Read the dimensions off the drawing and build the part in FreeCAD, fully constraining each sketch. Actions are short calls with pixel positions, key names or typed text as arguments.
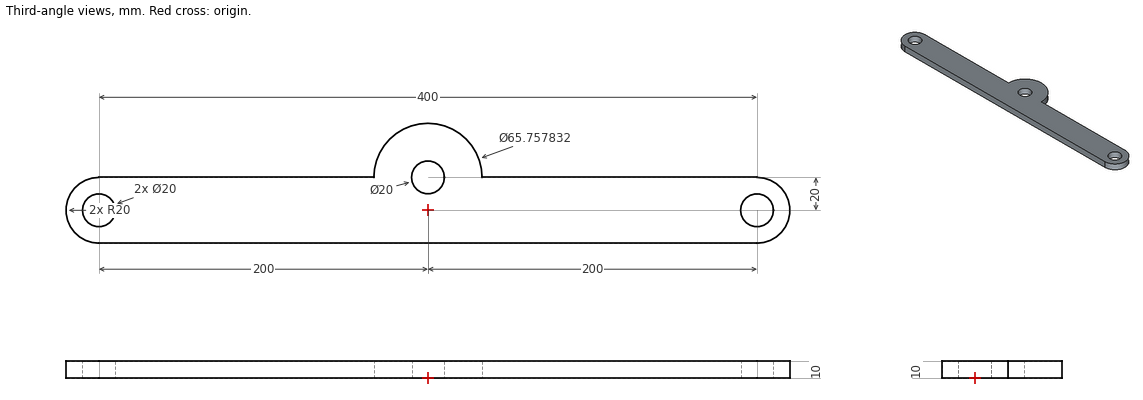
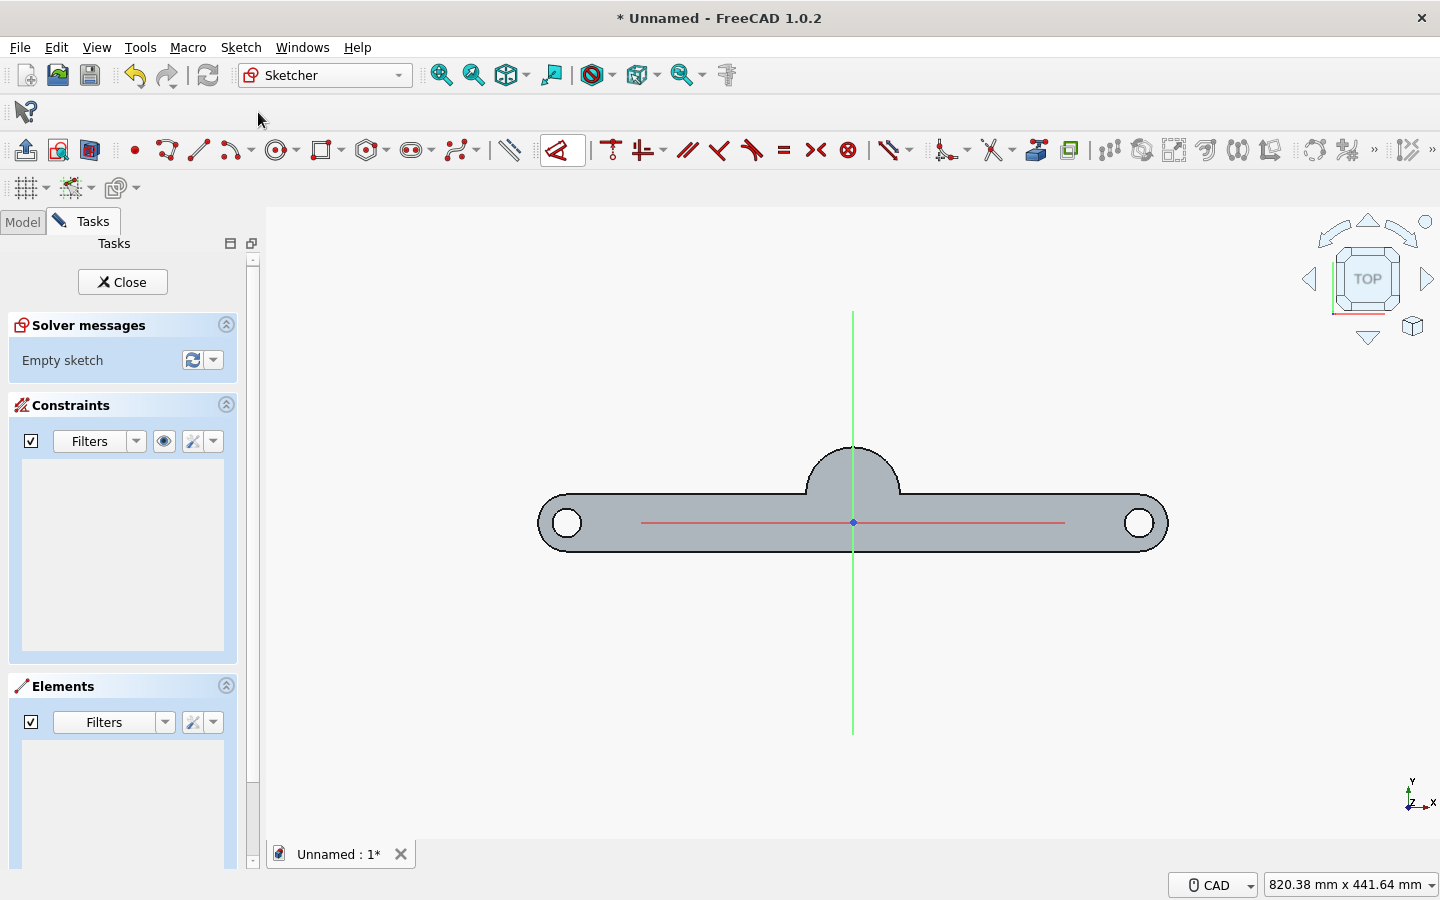
scroll(862, 499, up, 11)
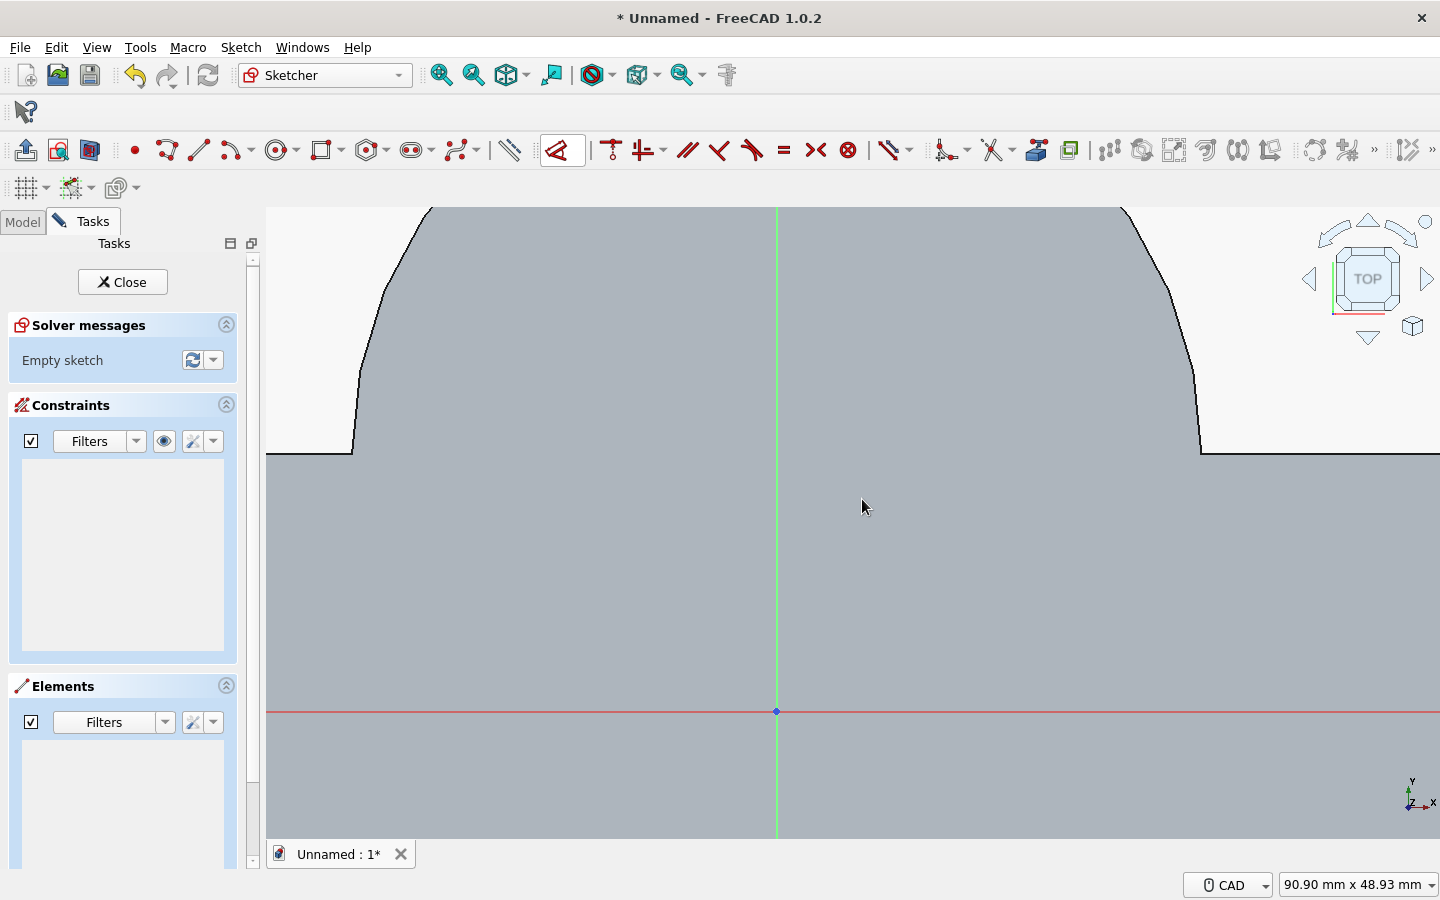
click(276, 150)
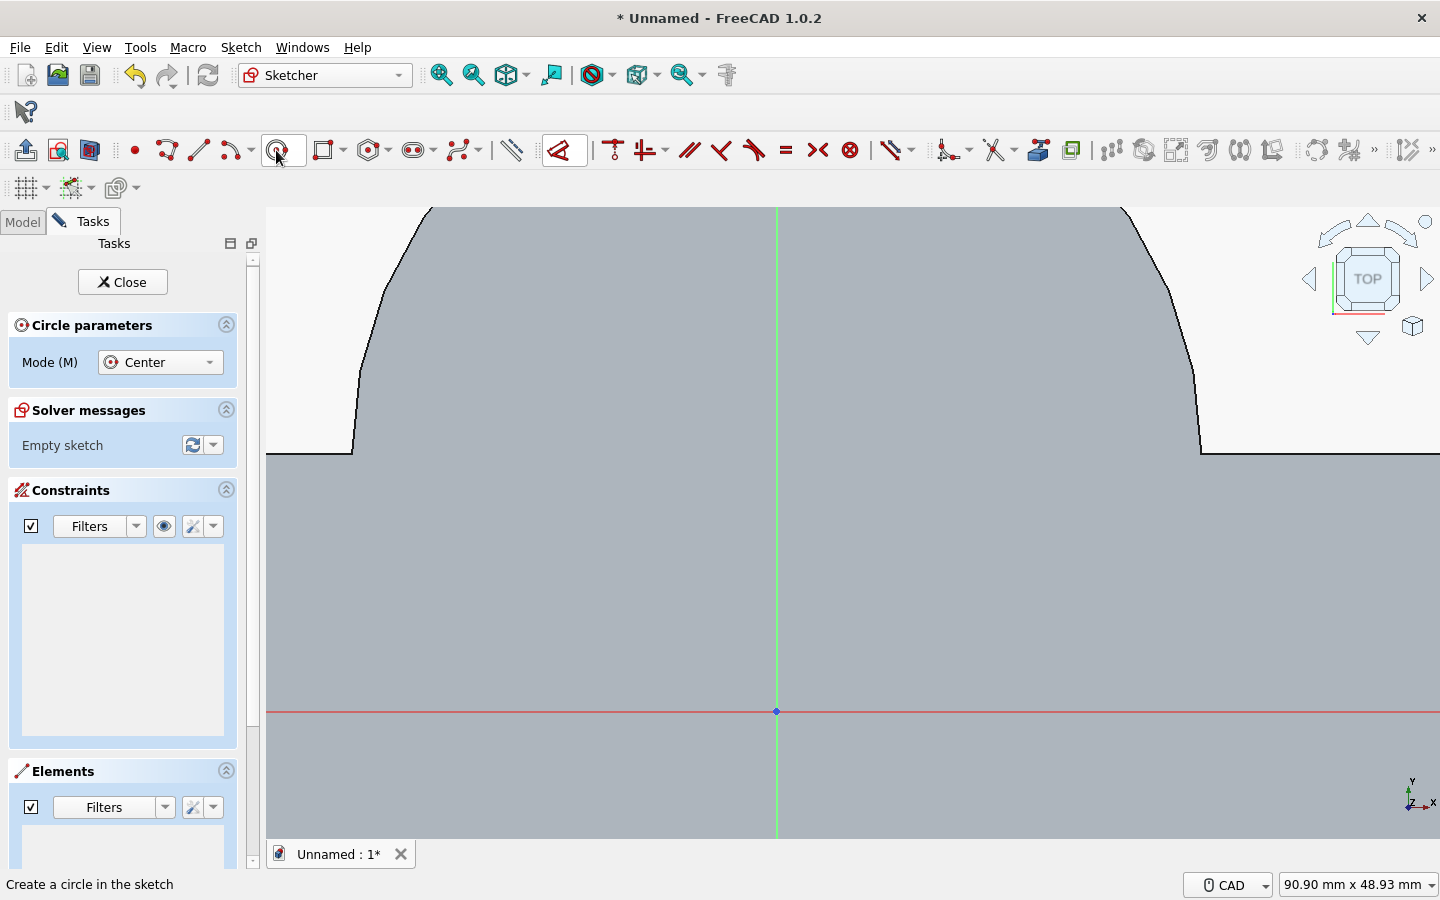
click(777, 454)
move(868, 362)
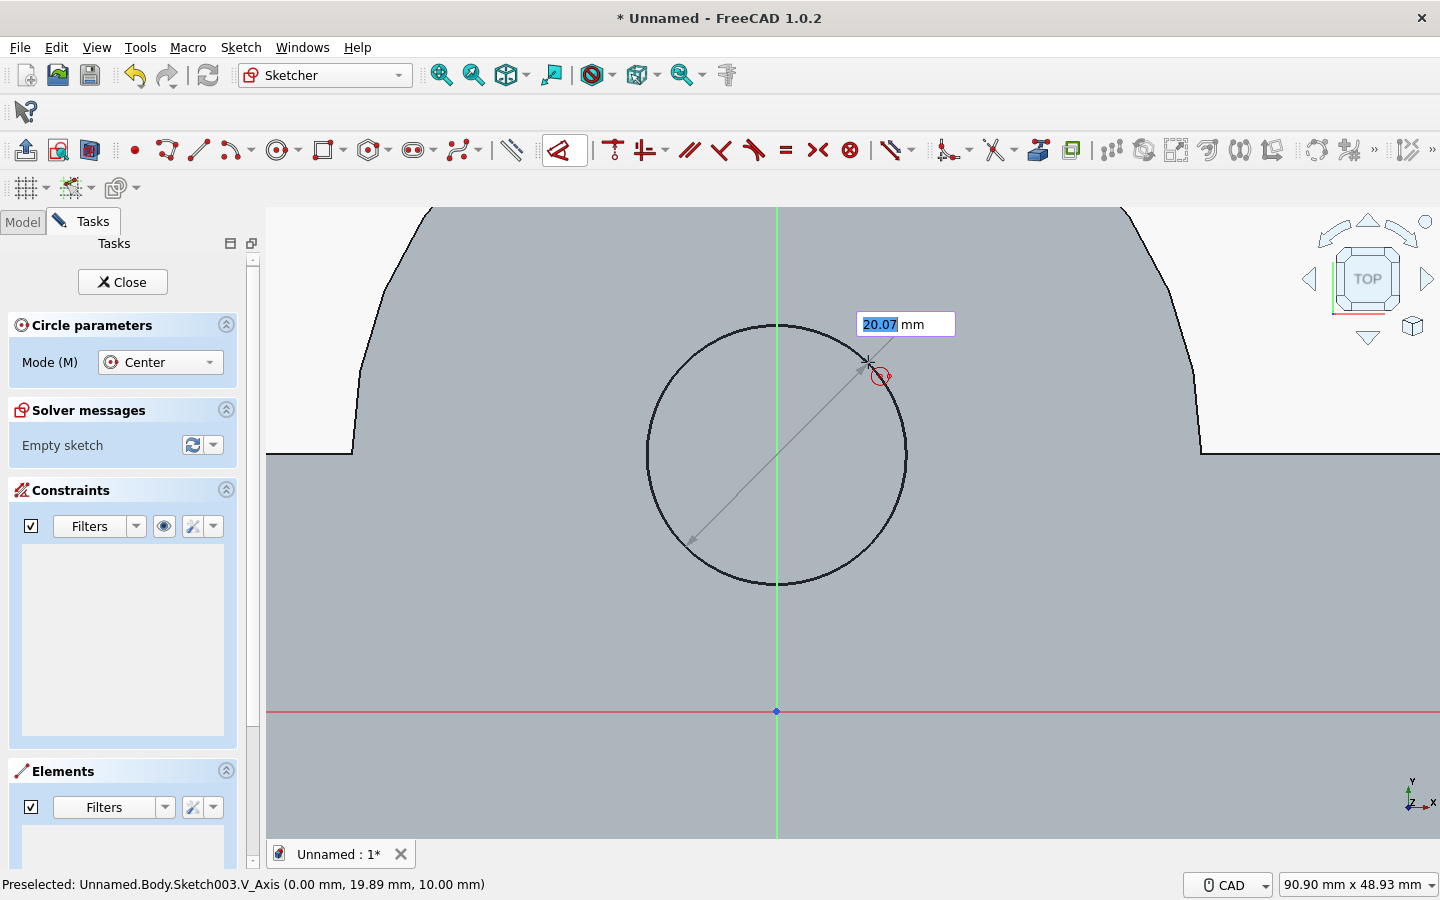
text(20)
key(Return)
key(Escape)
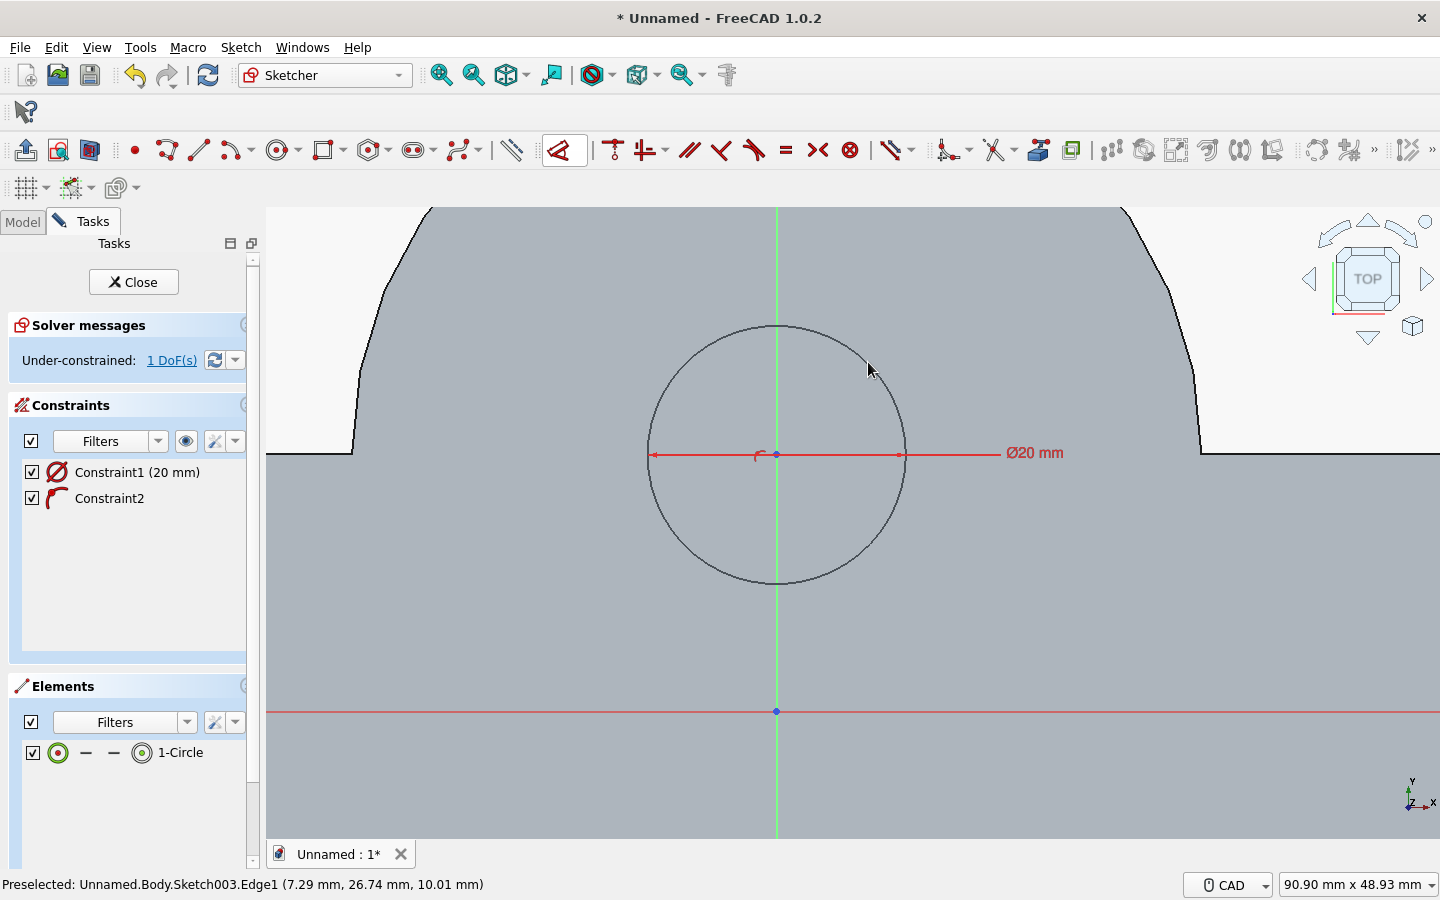
click(777, 455)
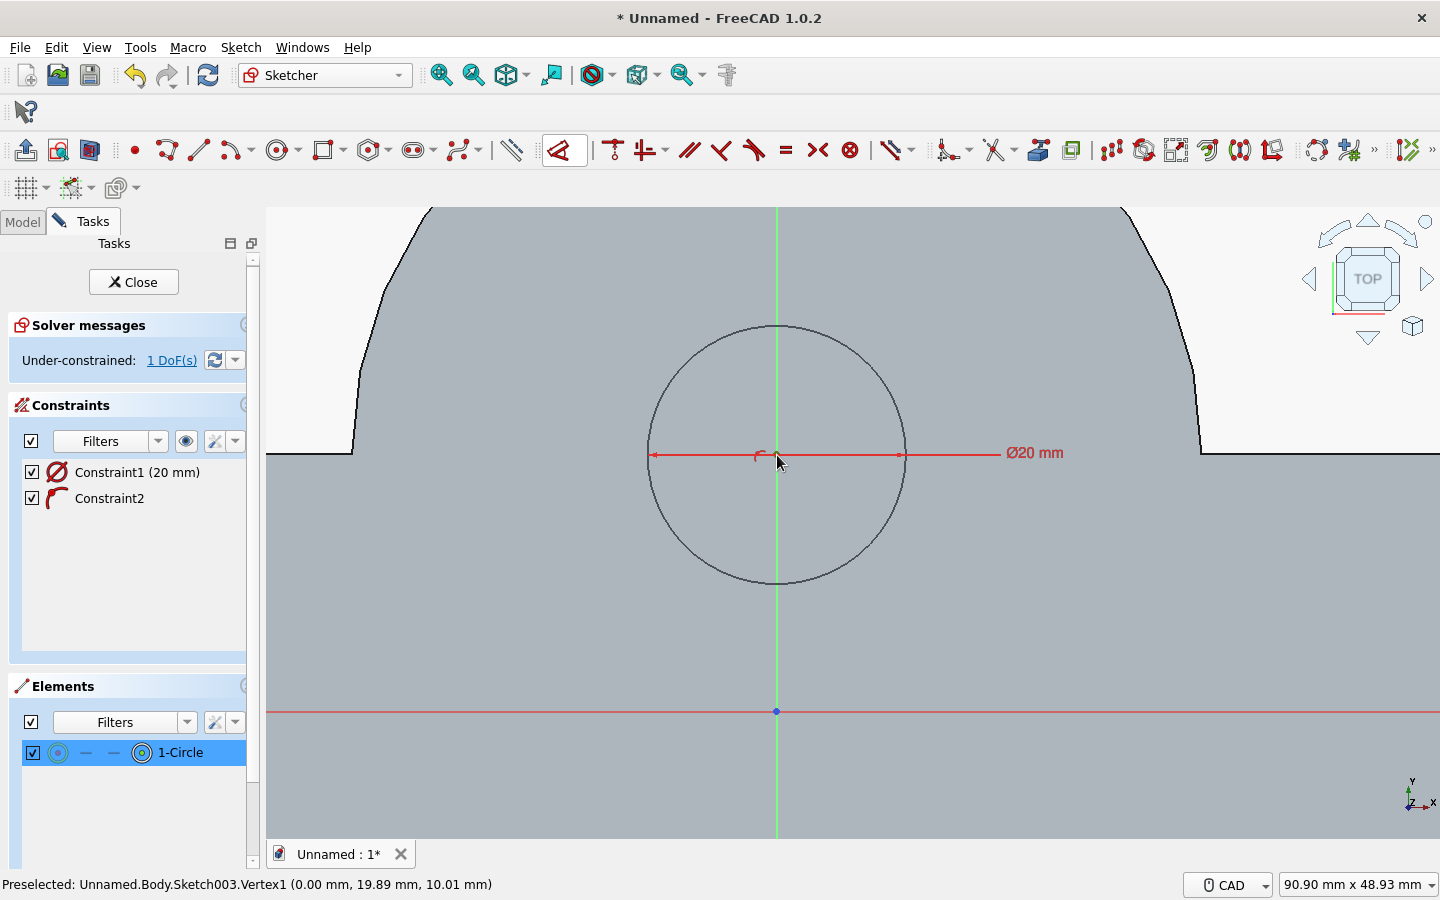
click(582, 150)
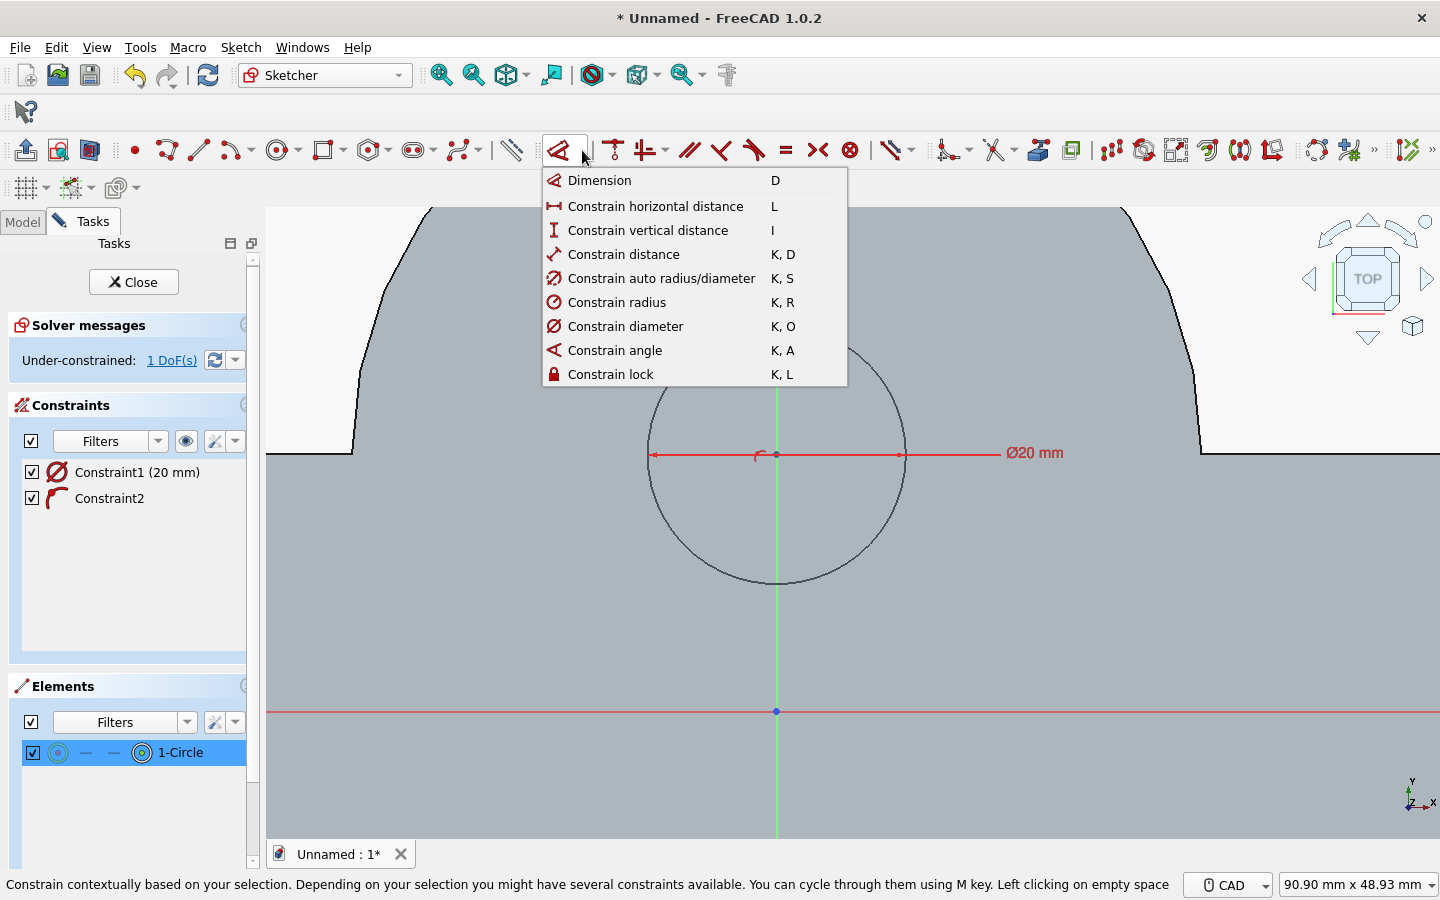
click(695, 230)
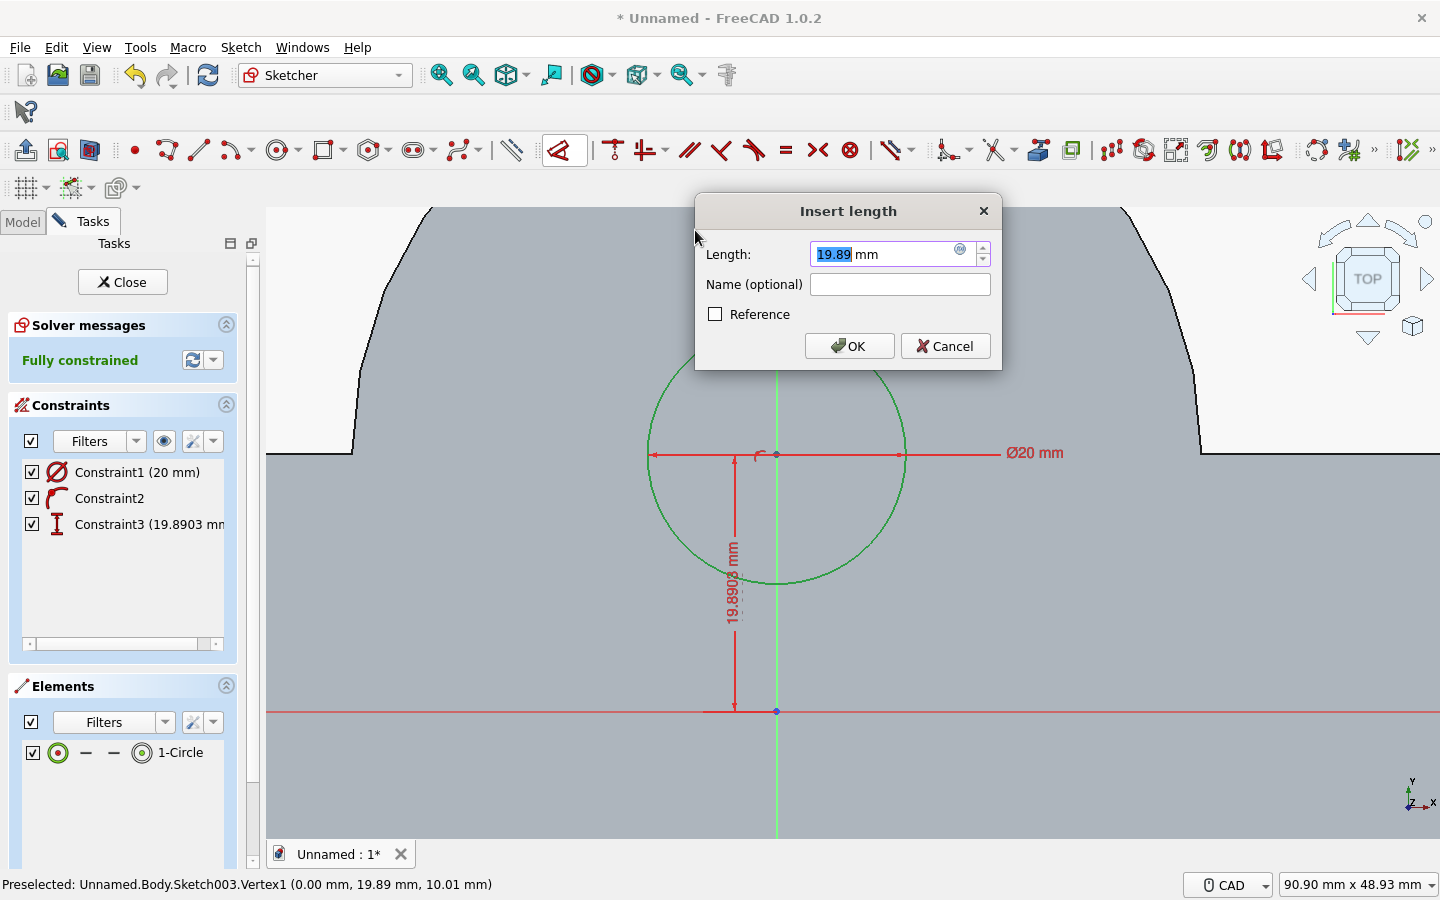
text(20)
key(Return)